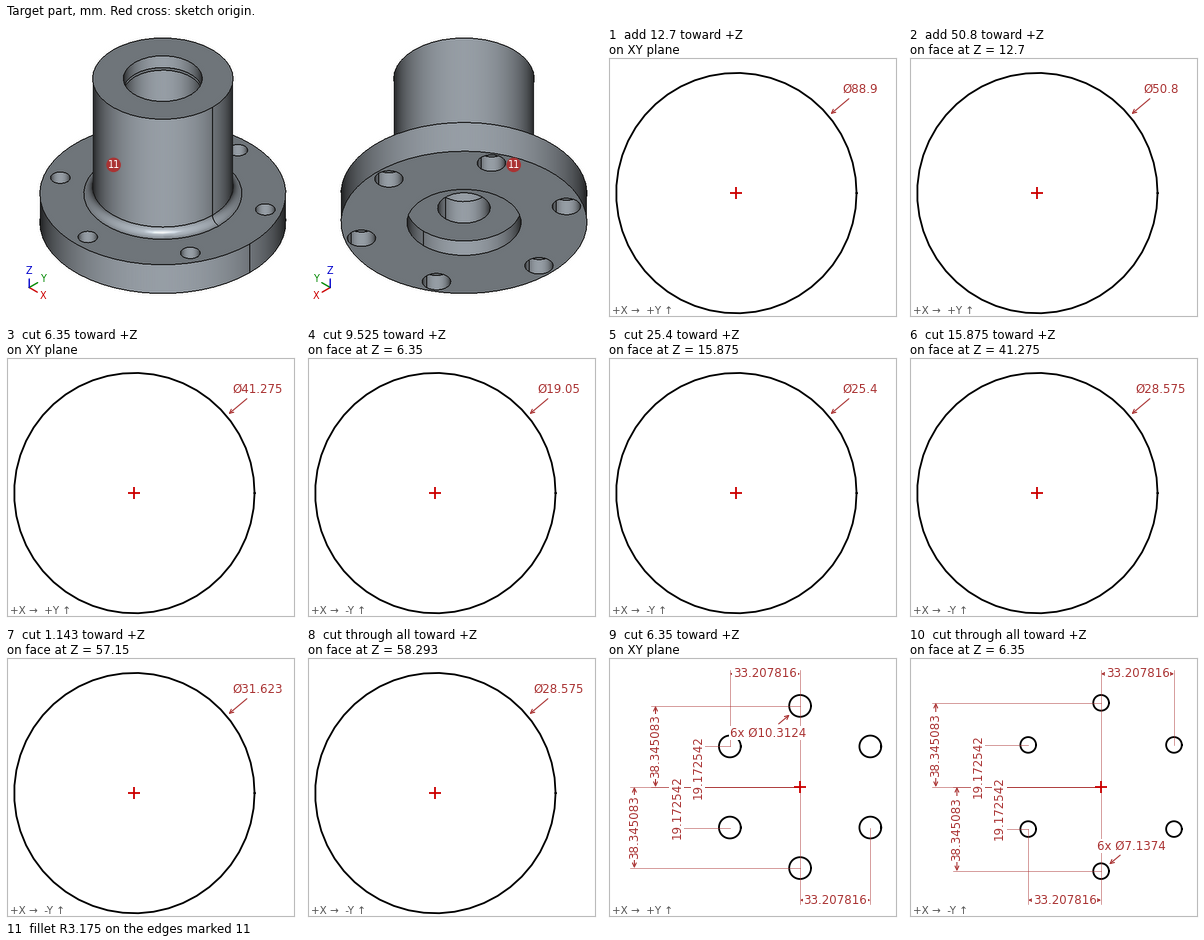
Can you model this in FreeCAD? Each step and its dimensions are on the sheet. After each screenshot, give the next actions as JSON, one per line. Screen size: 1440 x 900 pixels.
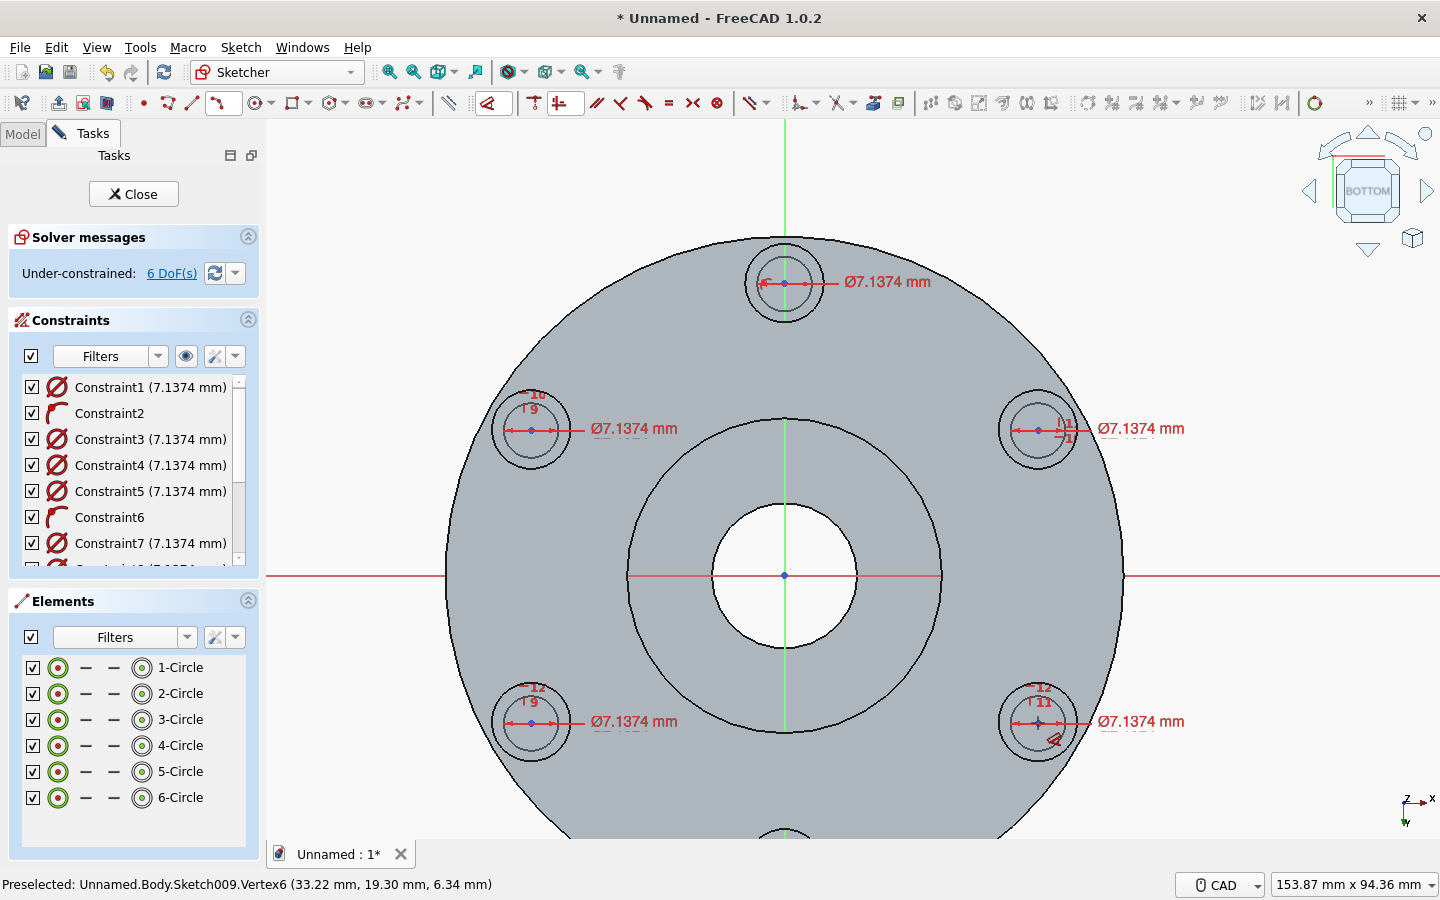
{"action": "scroll", "coordinate": [784, 282], "scroll_direction": "down", "scroll_amount": 2}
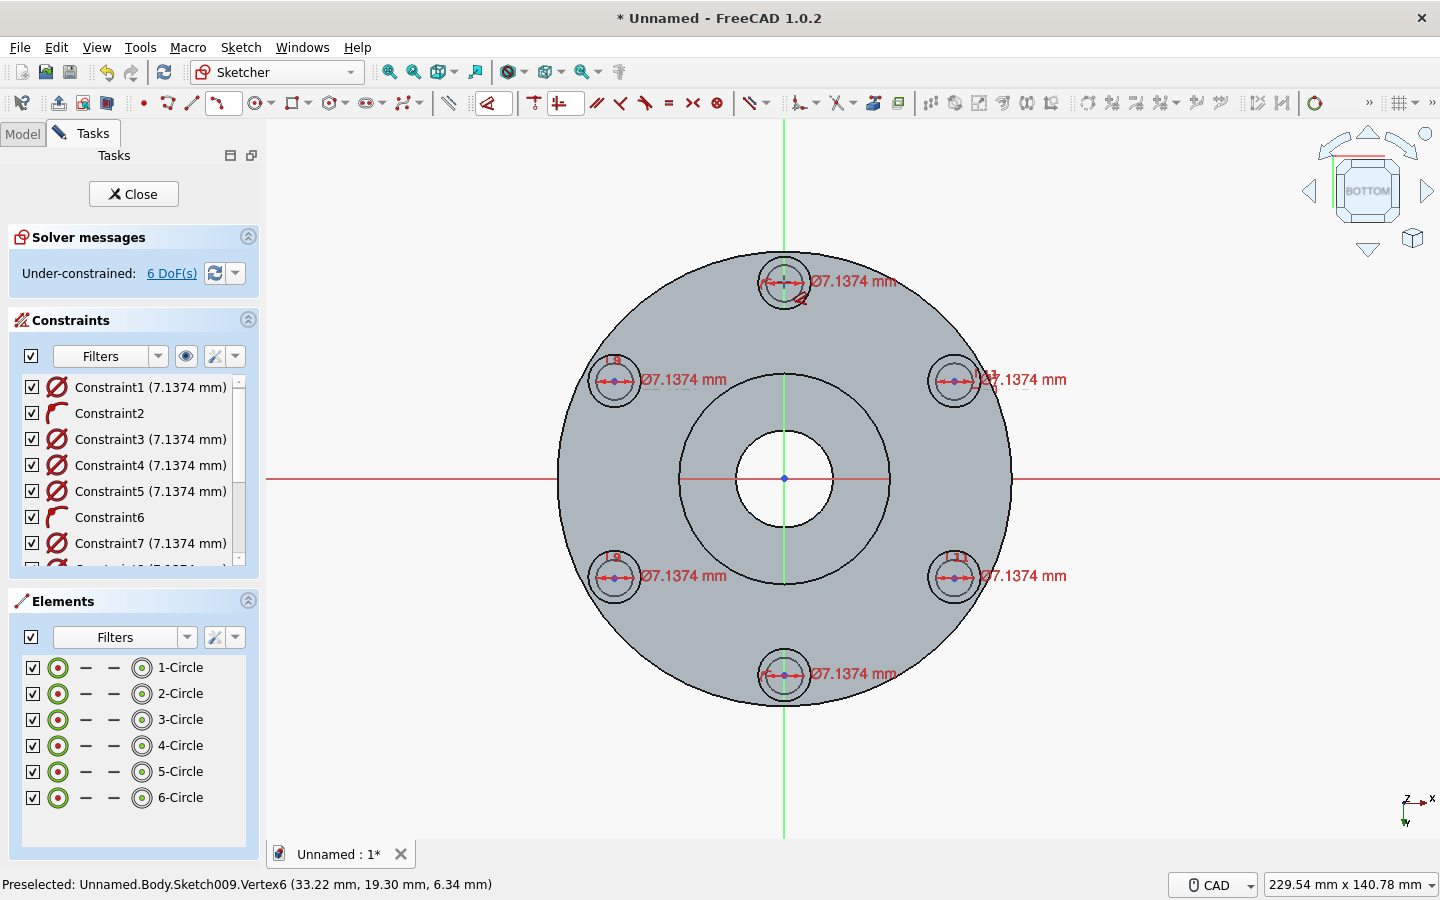
{"action": "left_click", "coordinate": [784, 676]}
{"action": "left_click", "coordinate": [818, 577]}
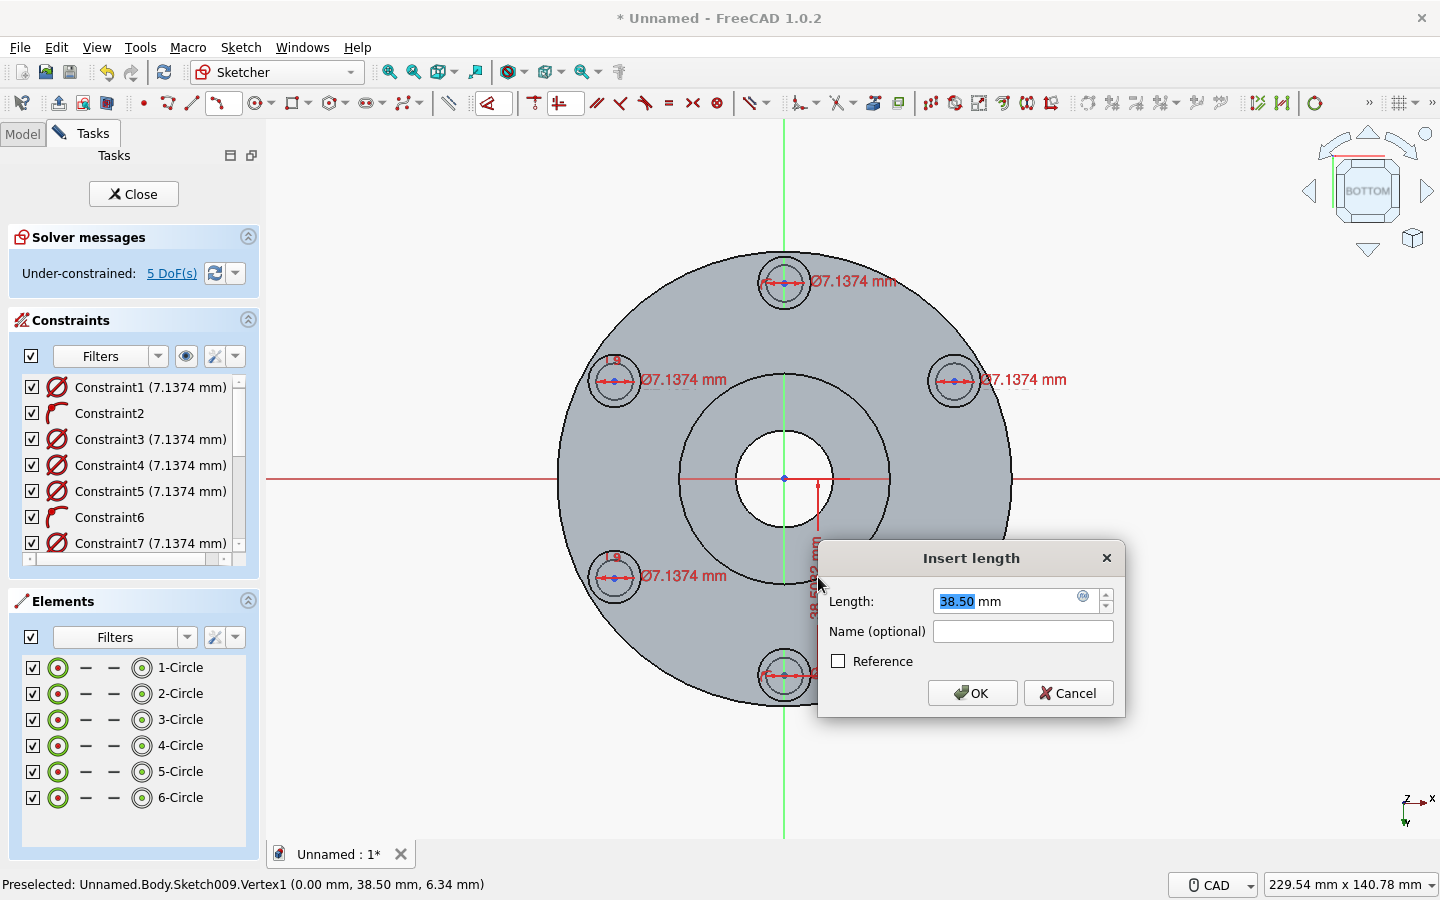
{"action": "type", "text": "38.345083"}
{"action": "key", "text": "Return"}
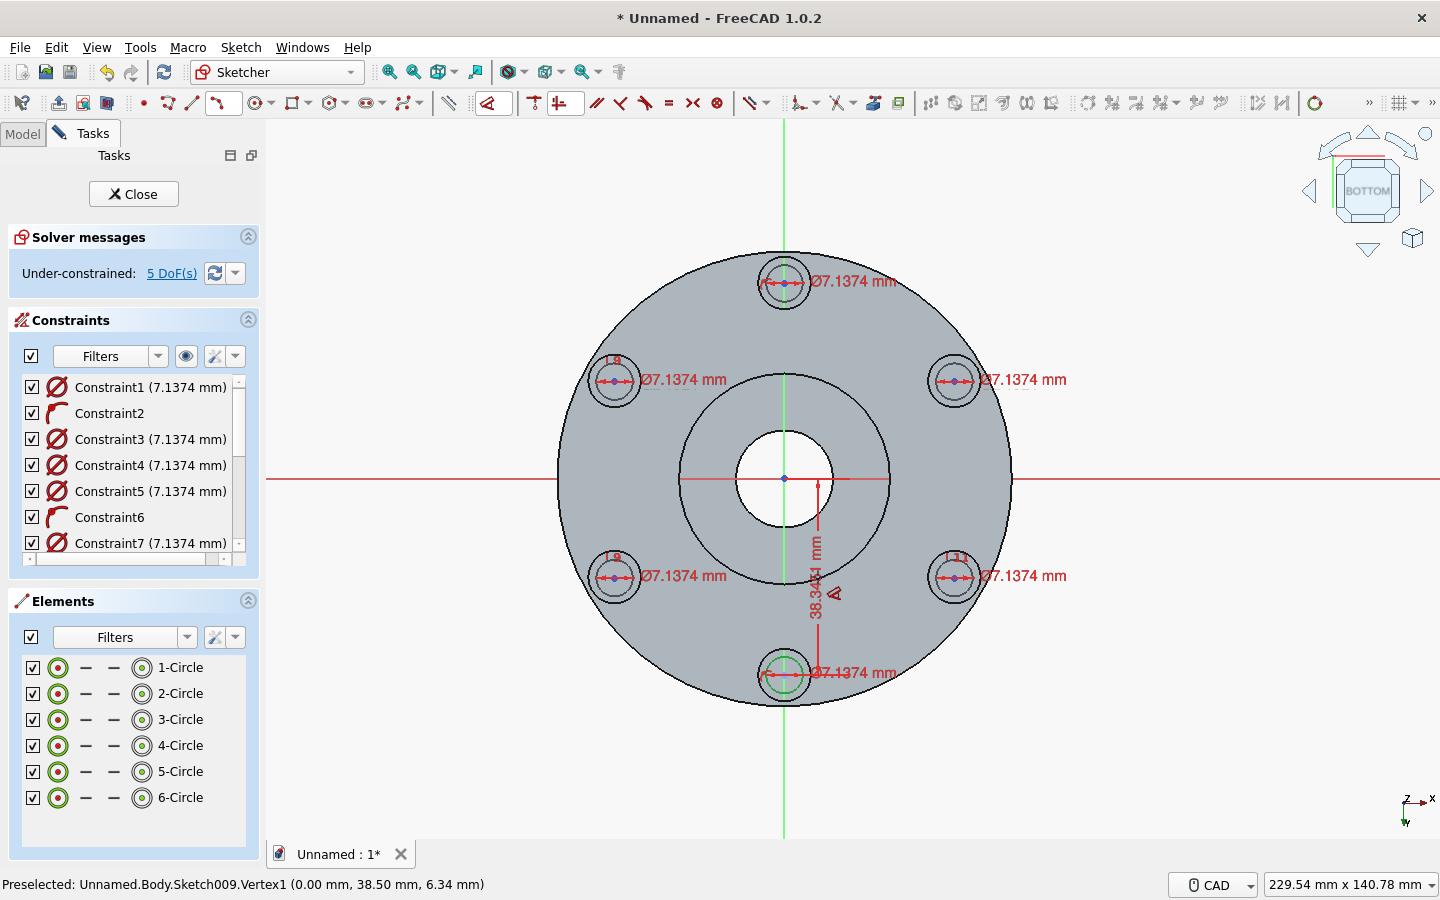
{"action": "left_click", "coordinate": [615, 578]}
{"action": "left_click", "coordinate": [700, 612]}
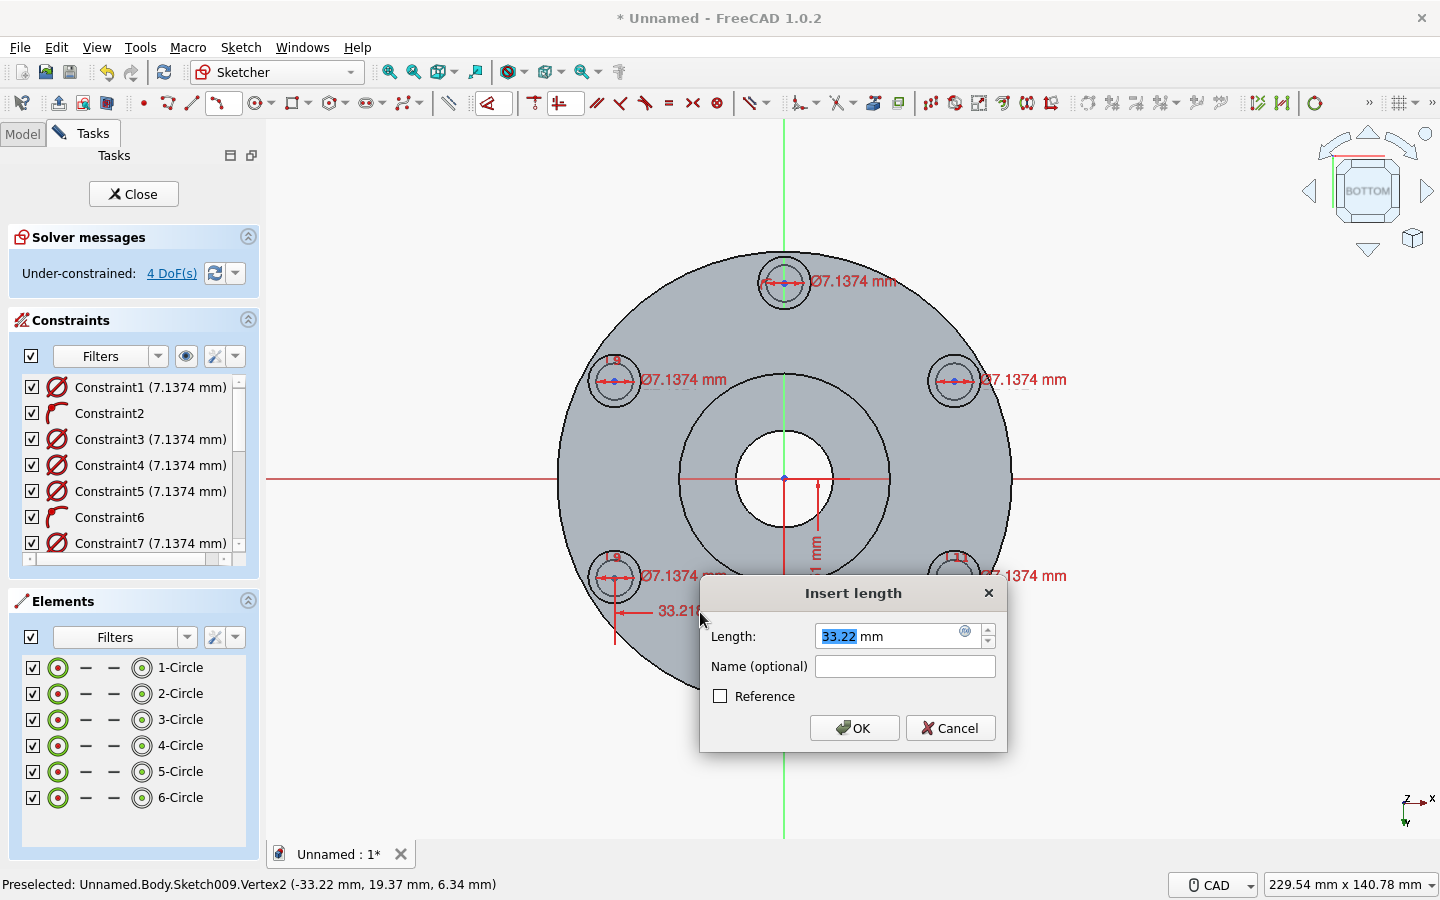
{"action": "type", "text": "33.207816"}
{"action": "key", "text": "Return"}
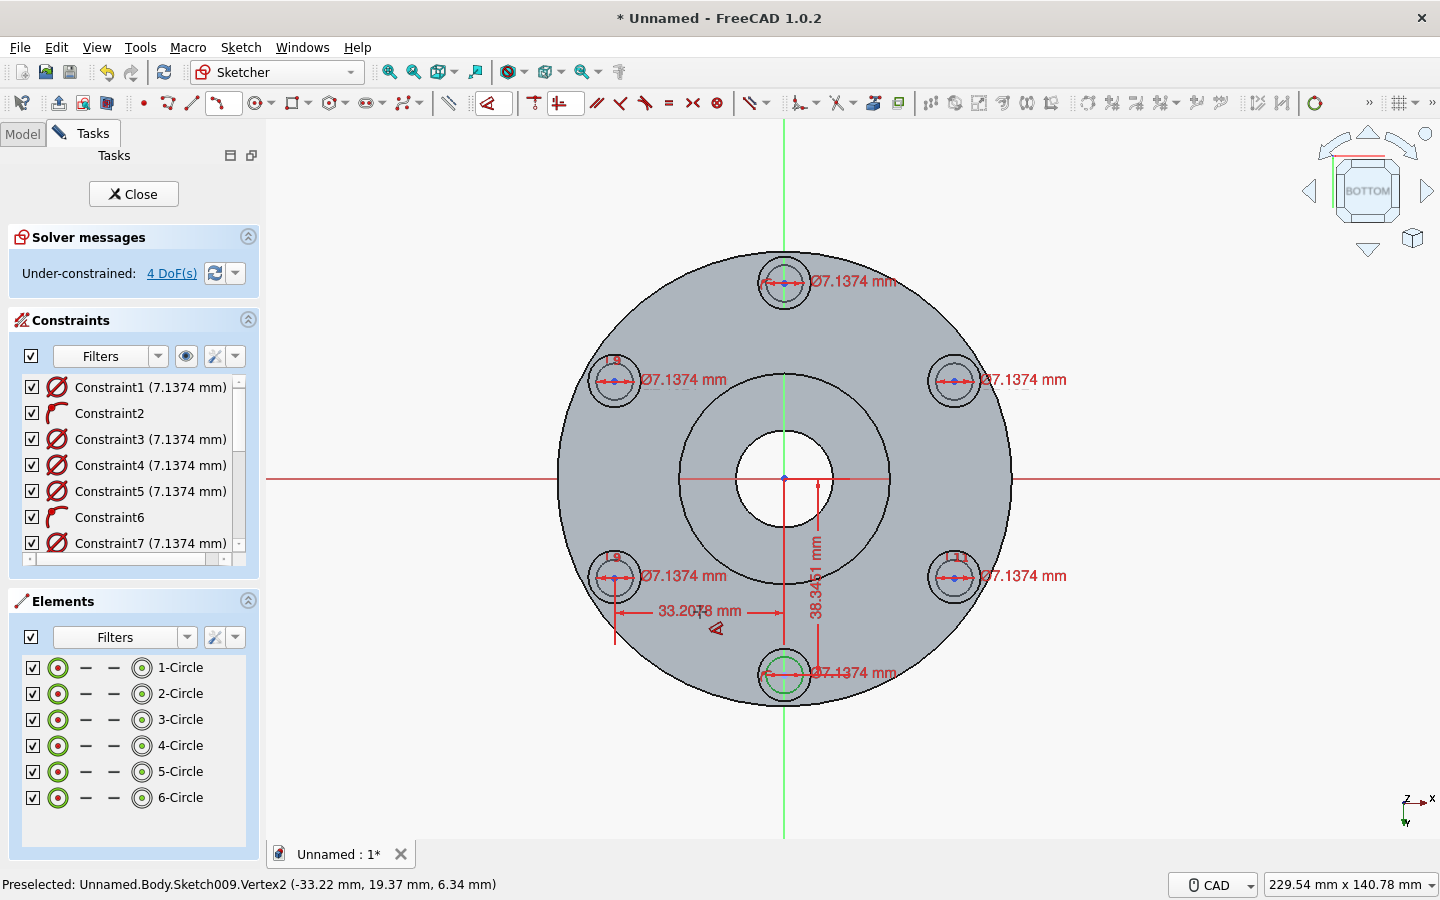
{"action": "left_click", "coordinate": [615, 578]}
{"action": "left_click", "coordinate": [581, 529]}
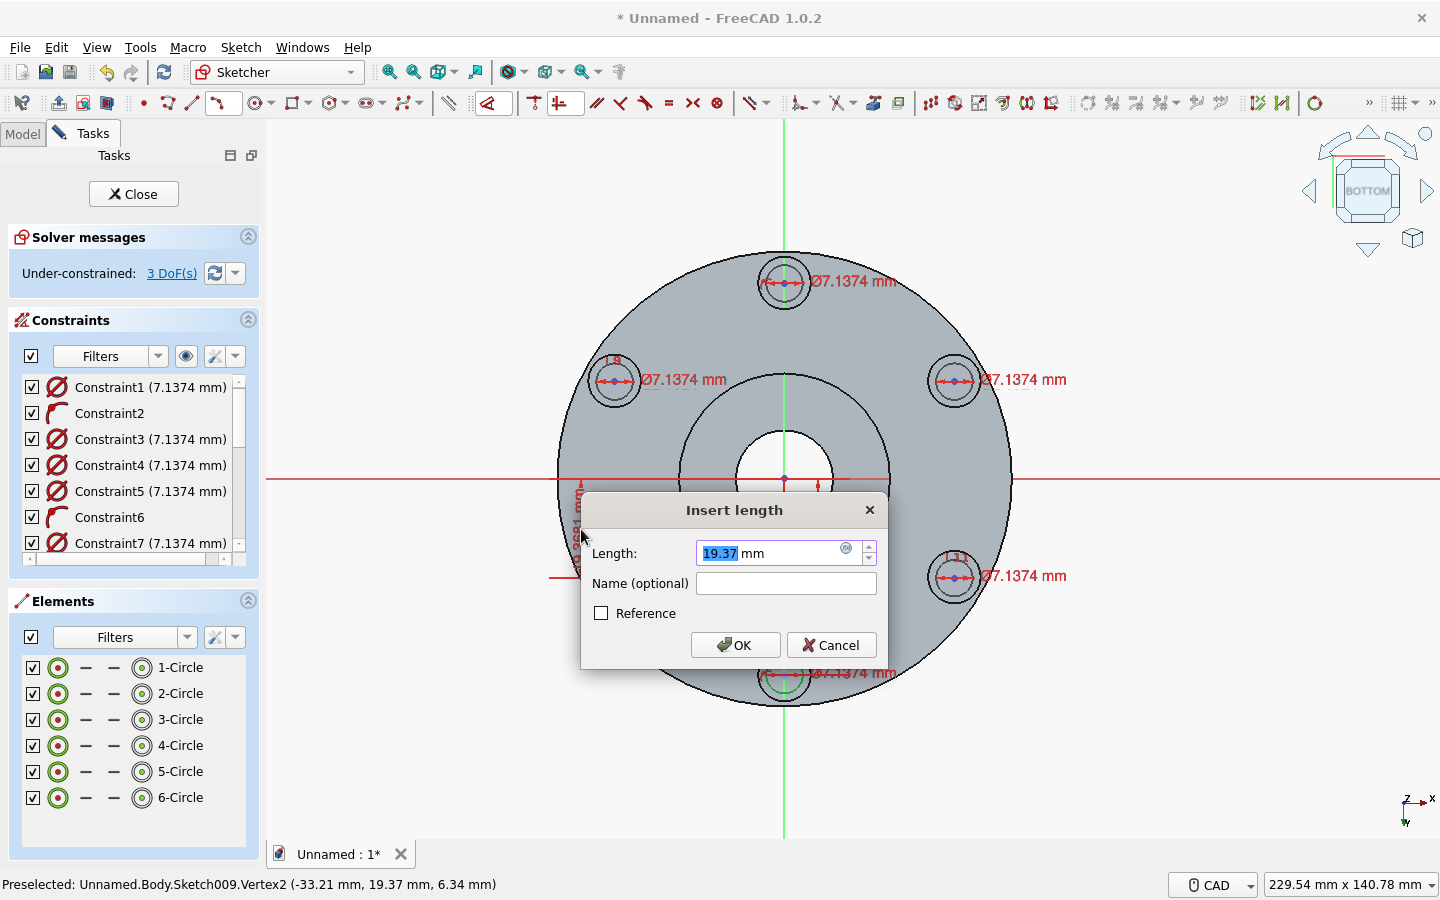
{"action": "type", "text": "19.172542"}
{"action": "key", "text": "Return"}